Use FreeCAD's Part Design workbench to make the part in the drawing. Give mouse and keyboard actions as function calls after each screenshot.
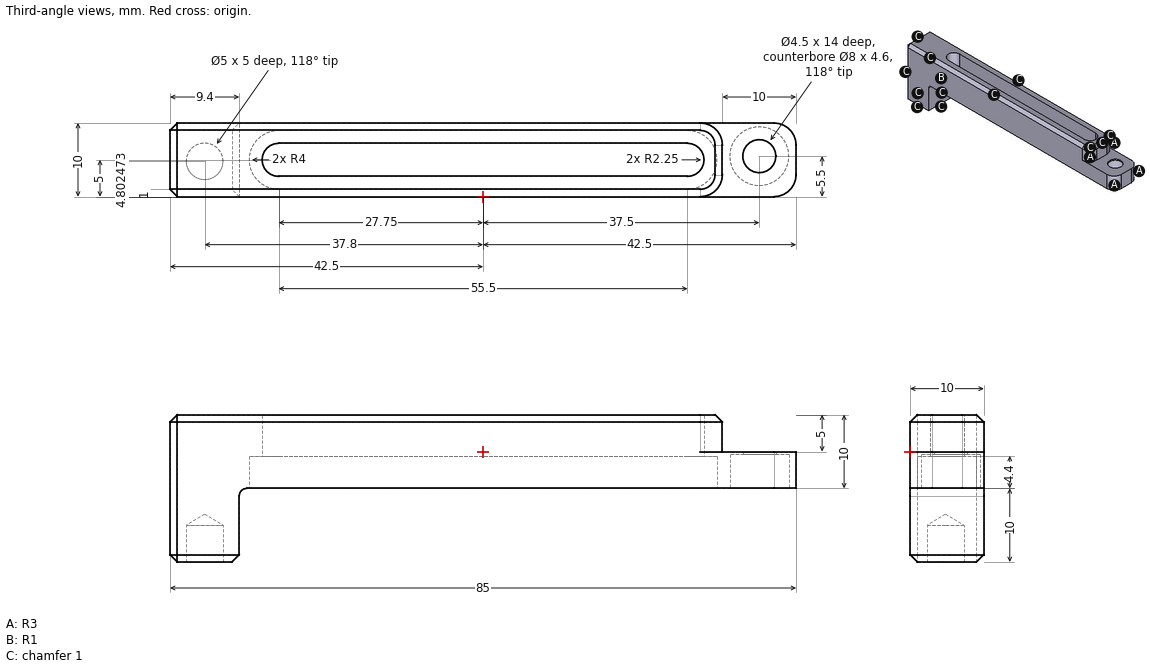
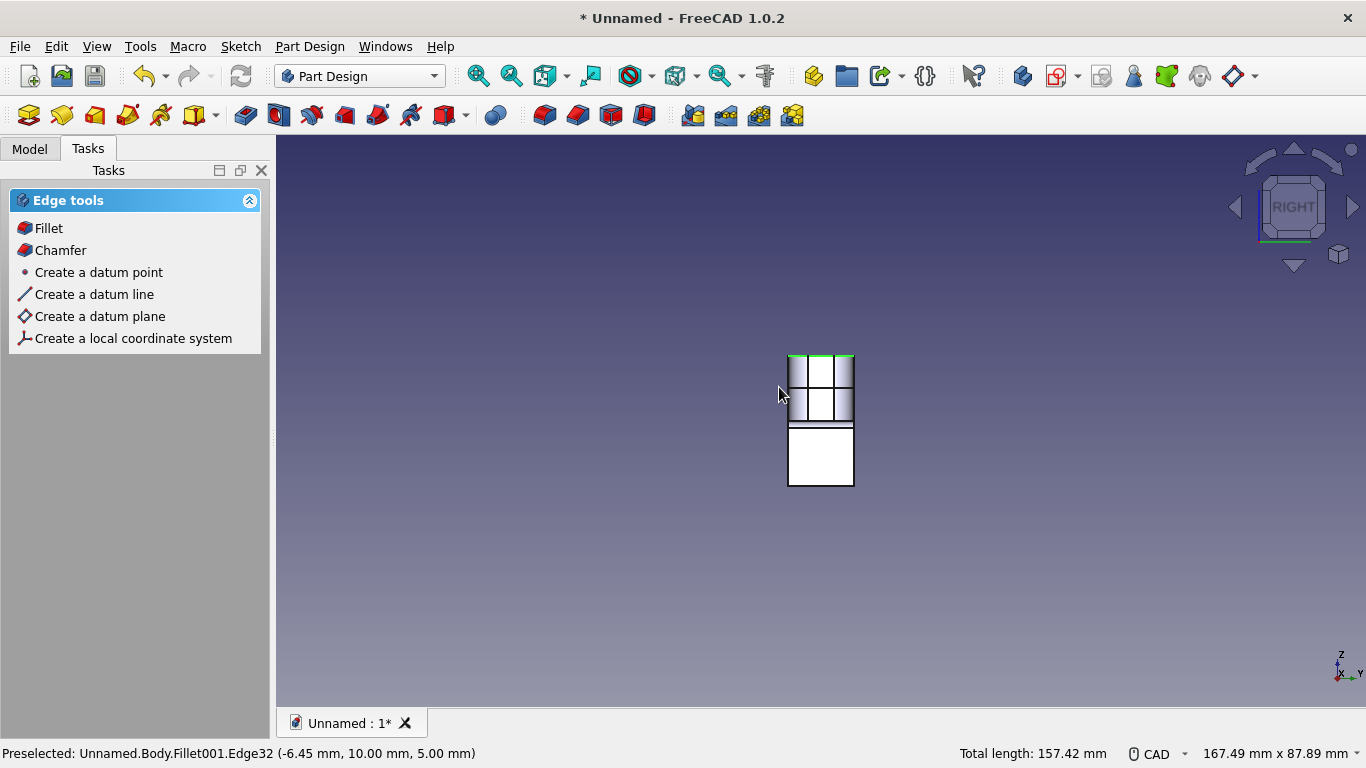
key(v)
key(f)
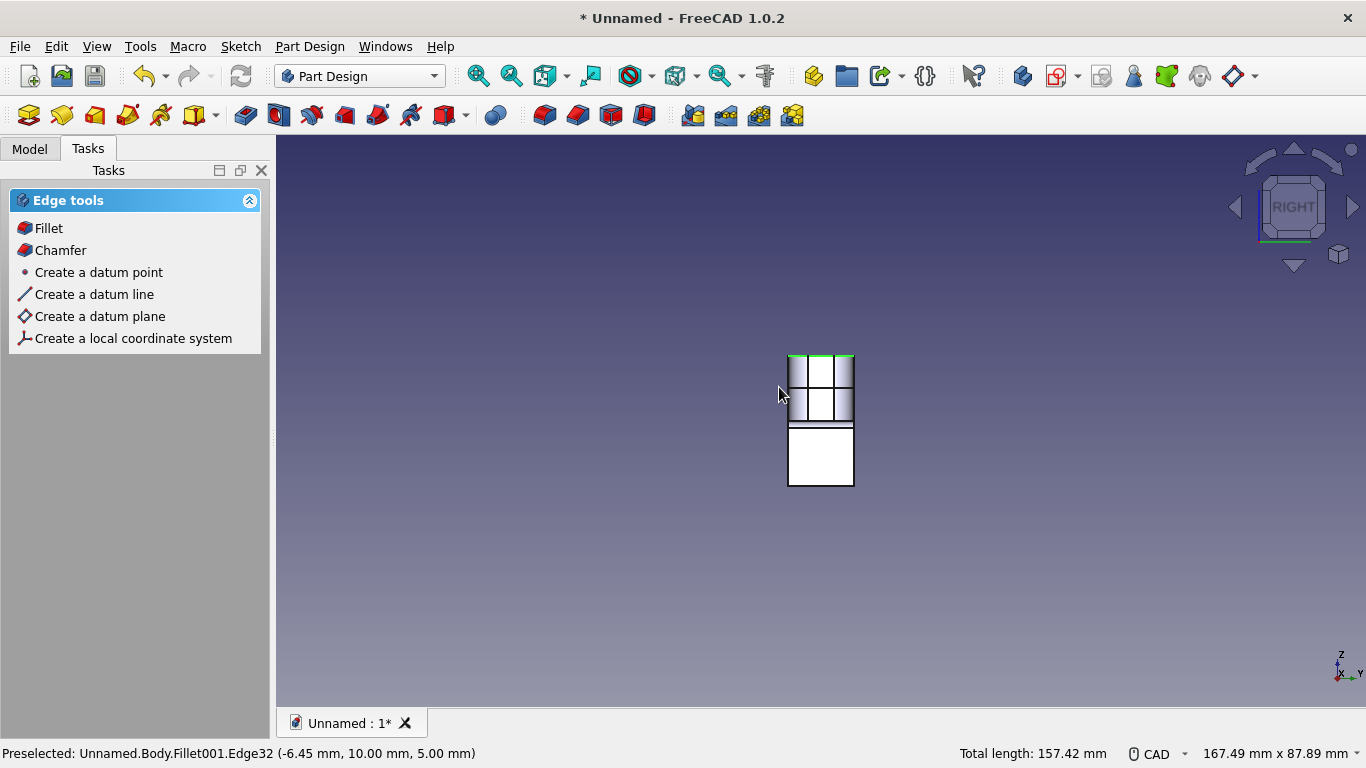
click(821, 485, ctrl)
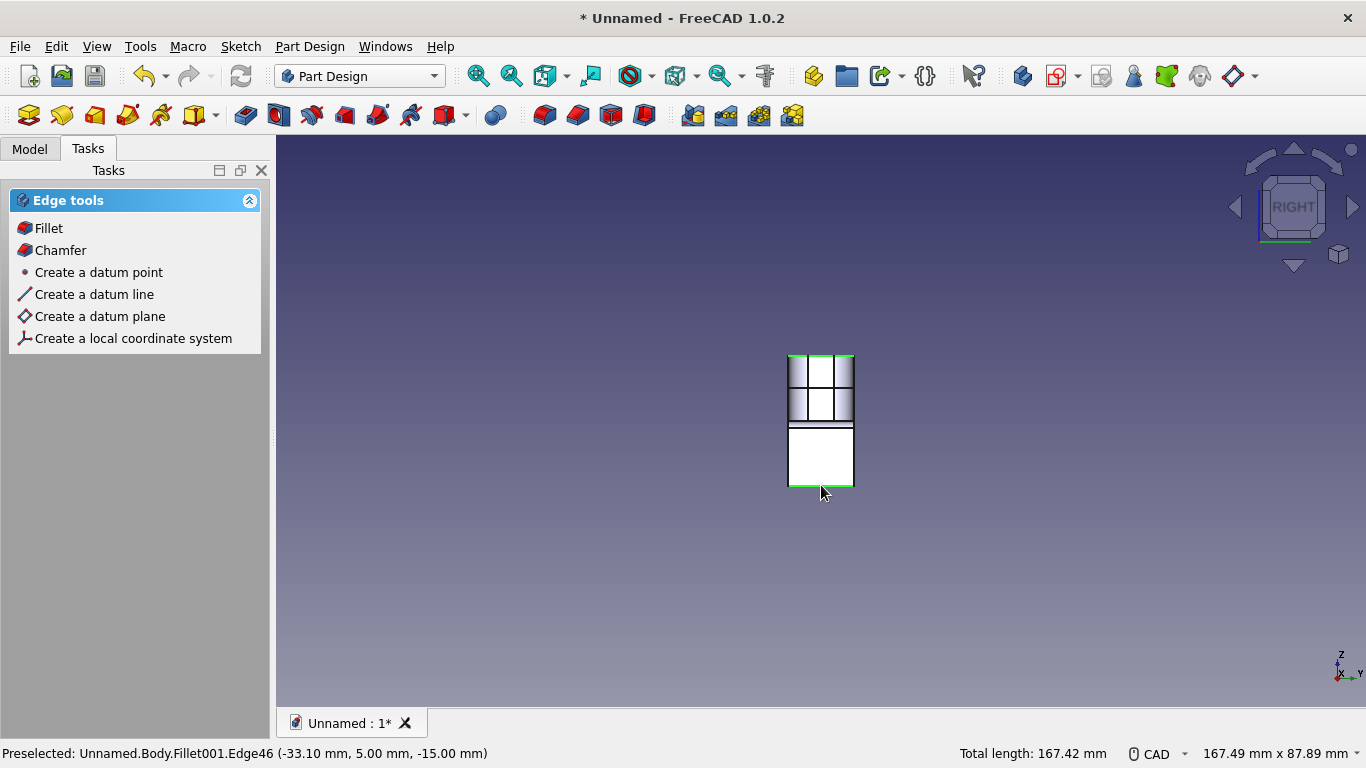
key(5)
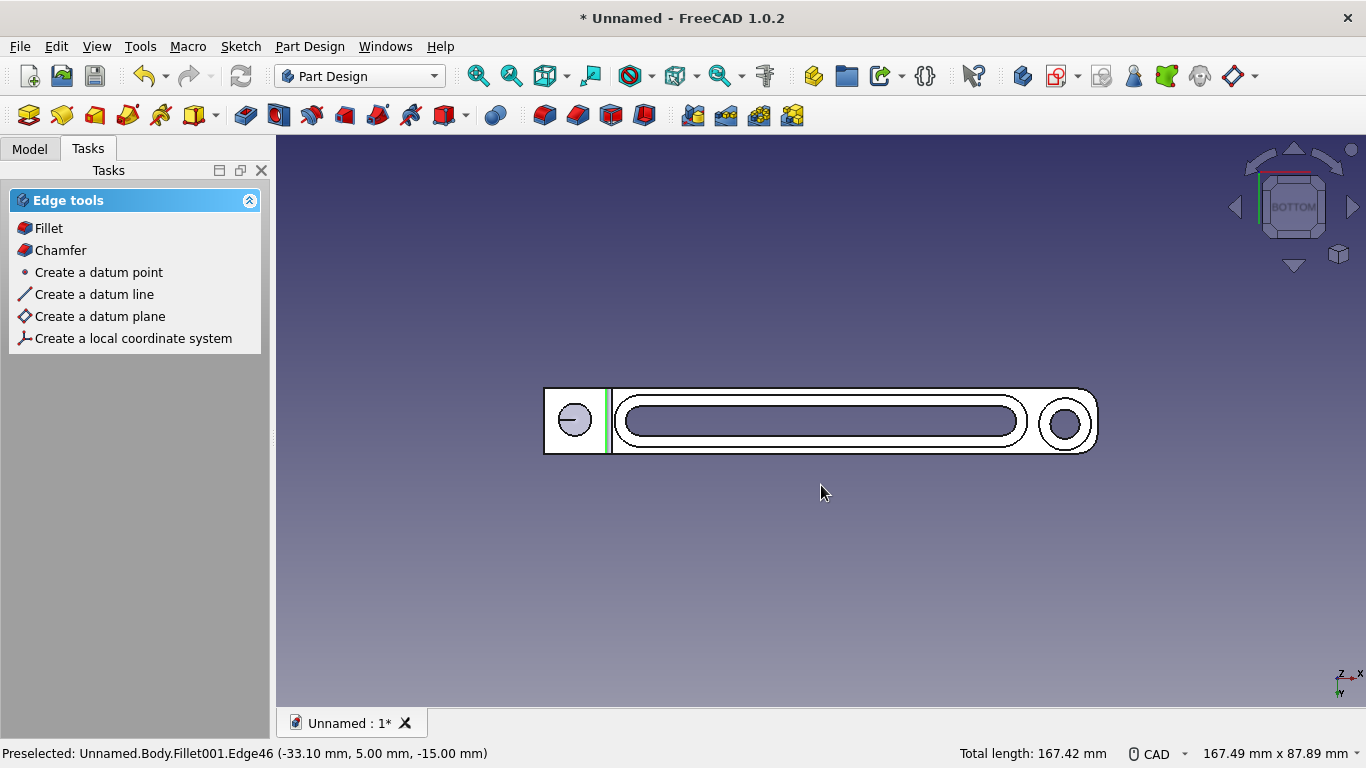
click(575, 387, ctrl)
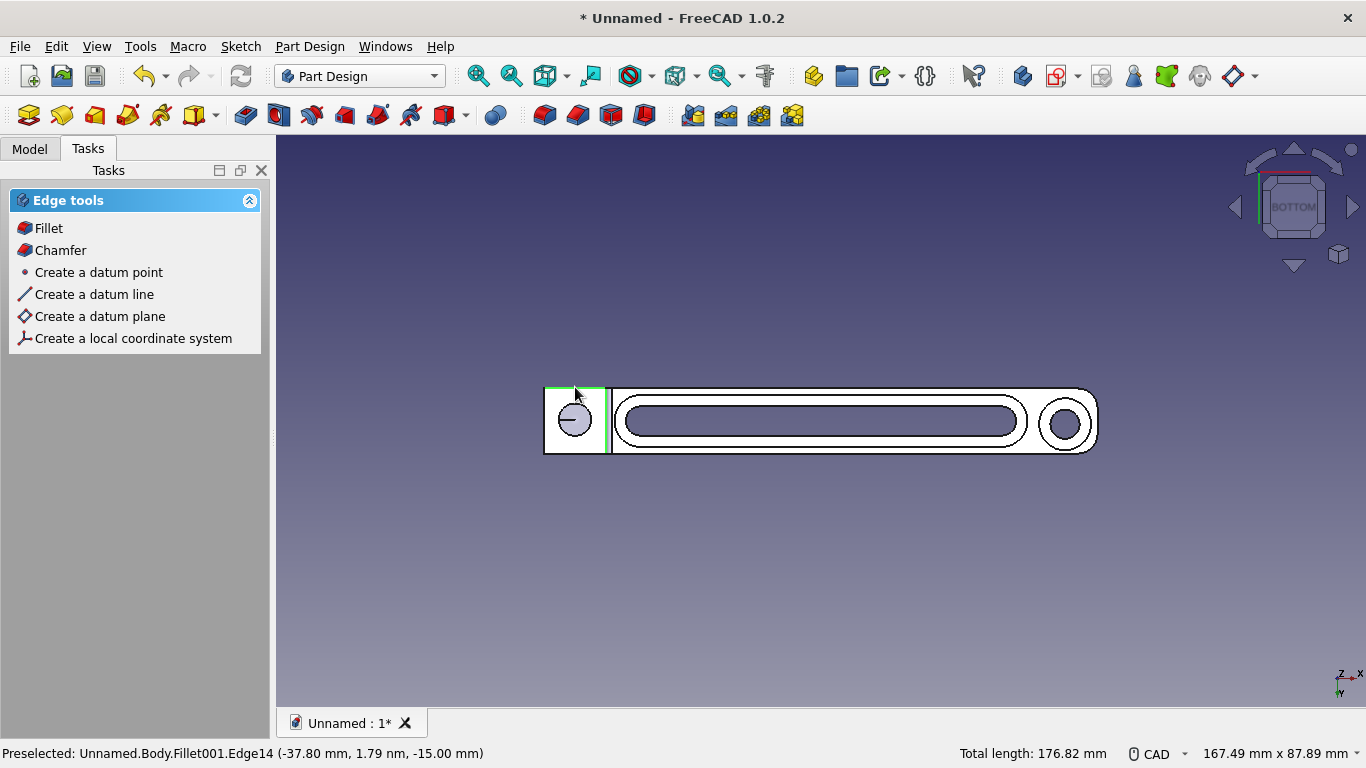
key(4)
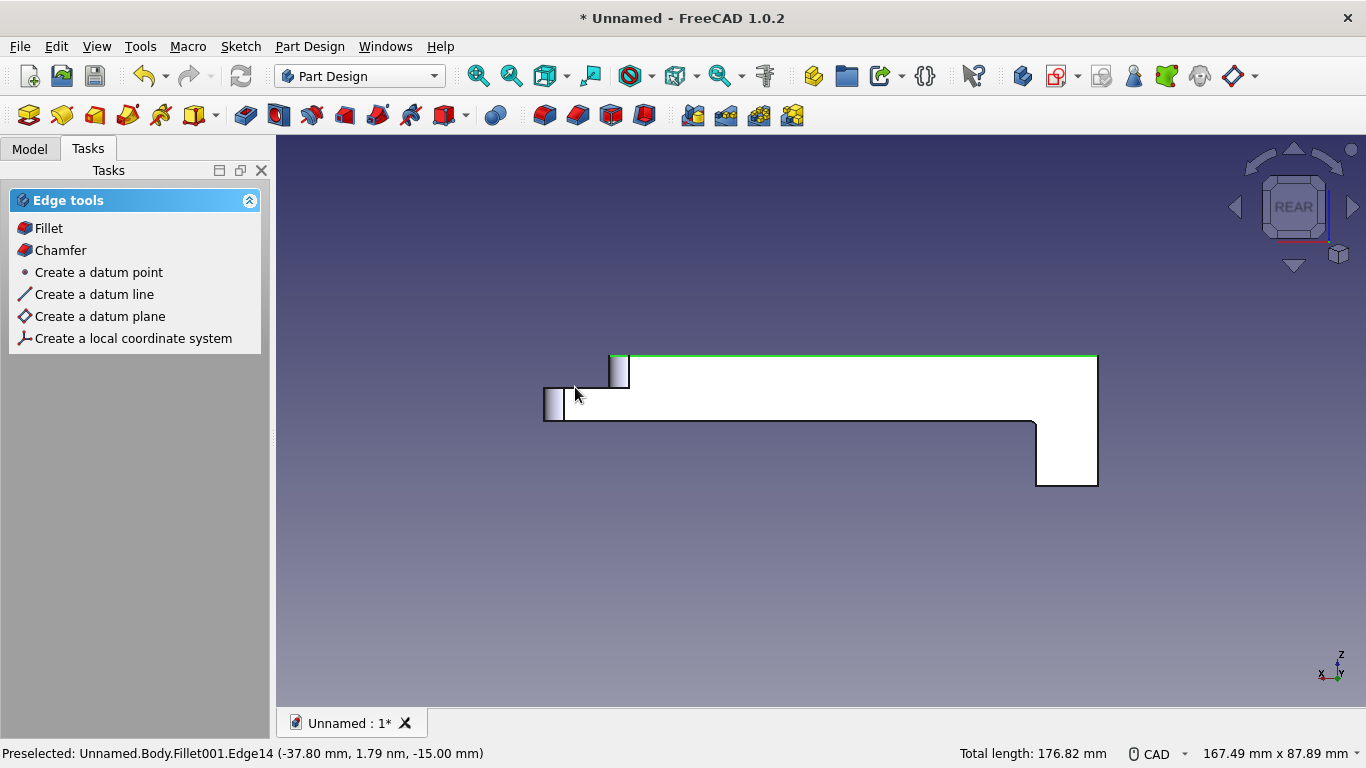
click(1067, 485, ctrl)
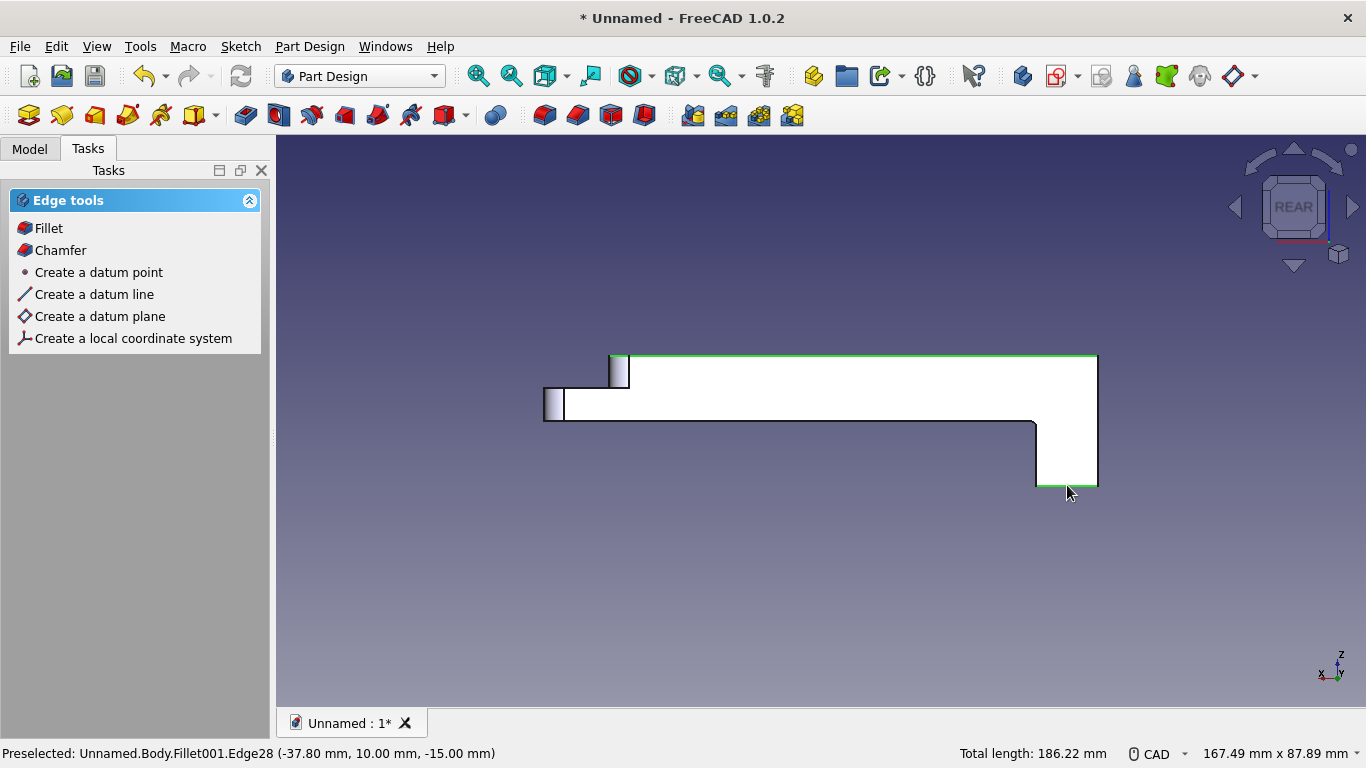
key(6)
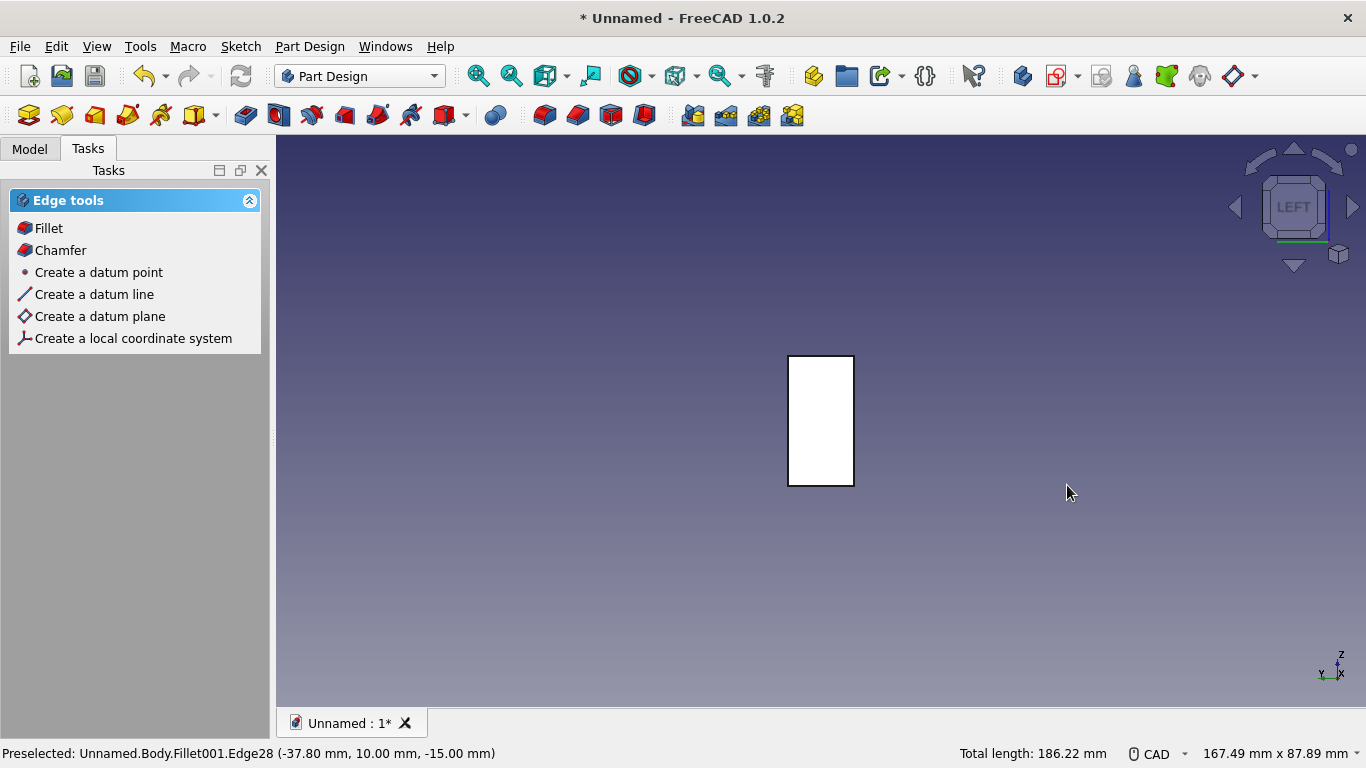
key(v)
key(f)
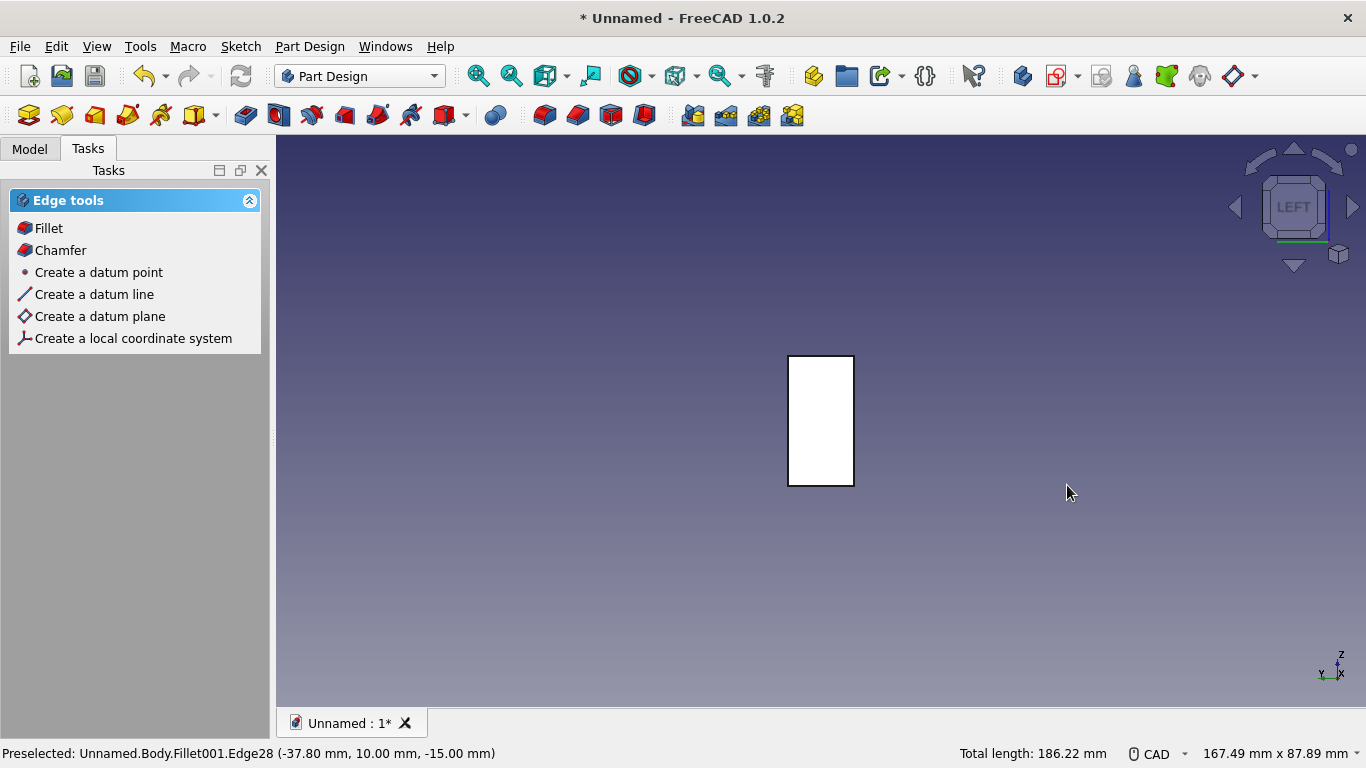
click(821, 439, ctrl)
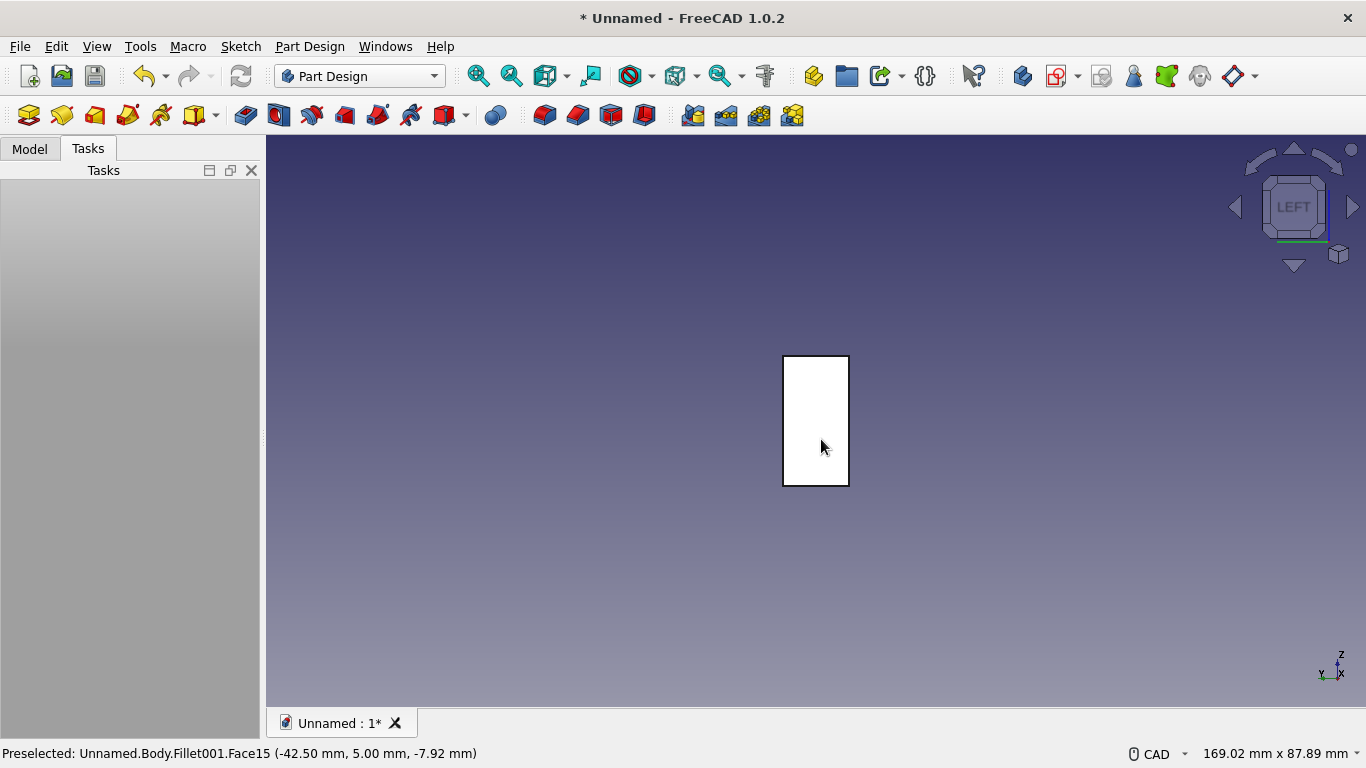
click(578, 116)